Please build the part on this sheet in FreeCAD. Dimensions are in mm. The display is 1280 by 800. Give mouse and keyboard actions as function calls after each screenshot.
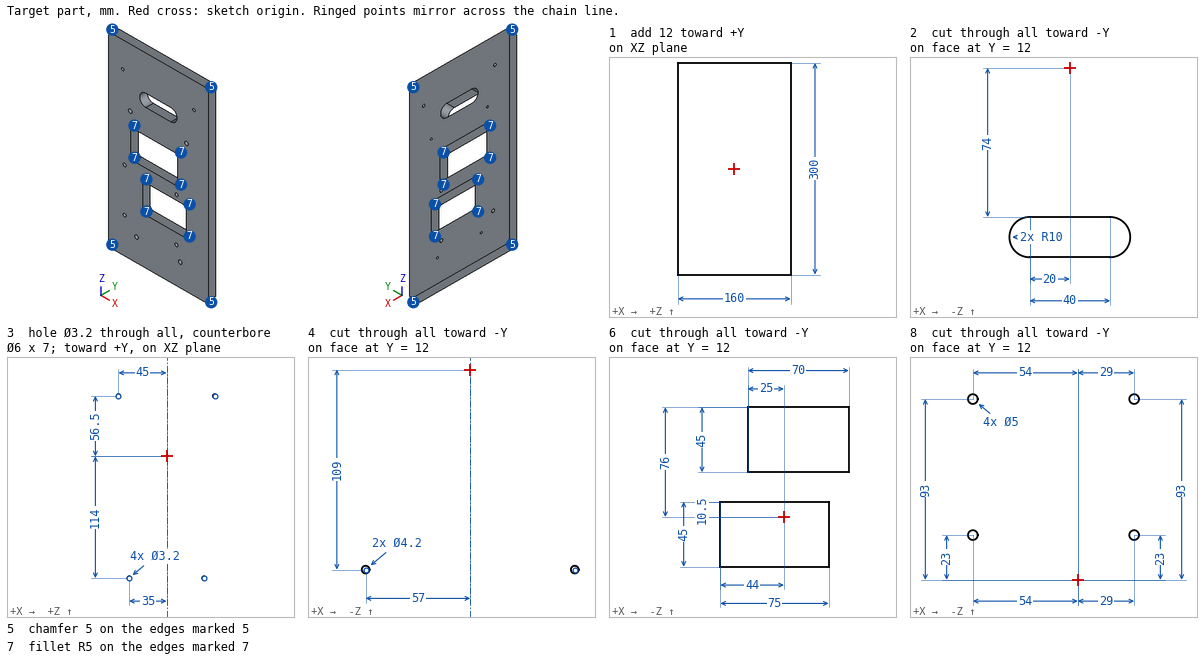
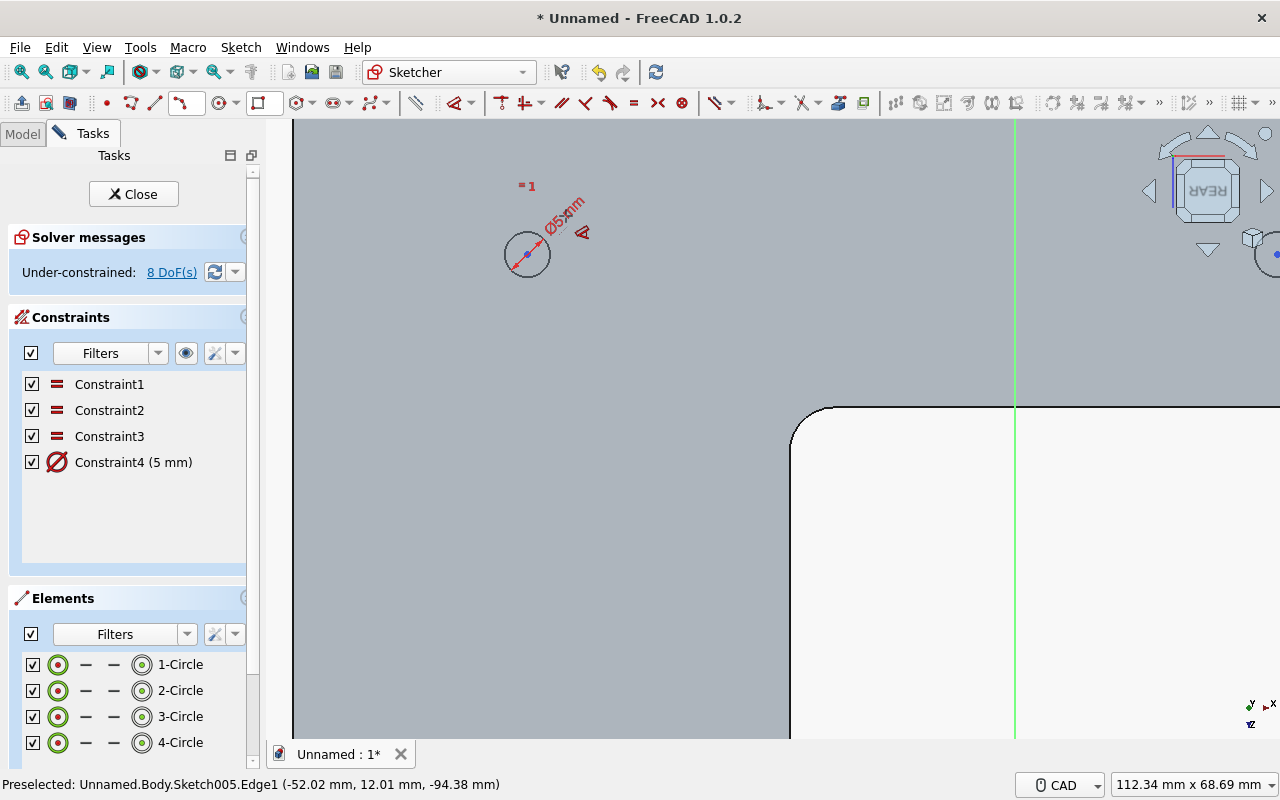
click(527, 255)
click(771, 221)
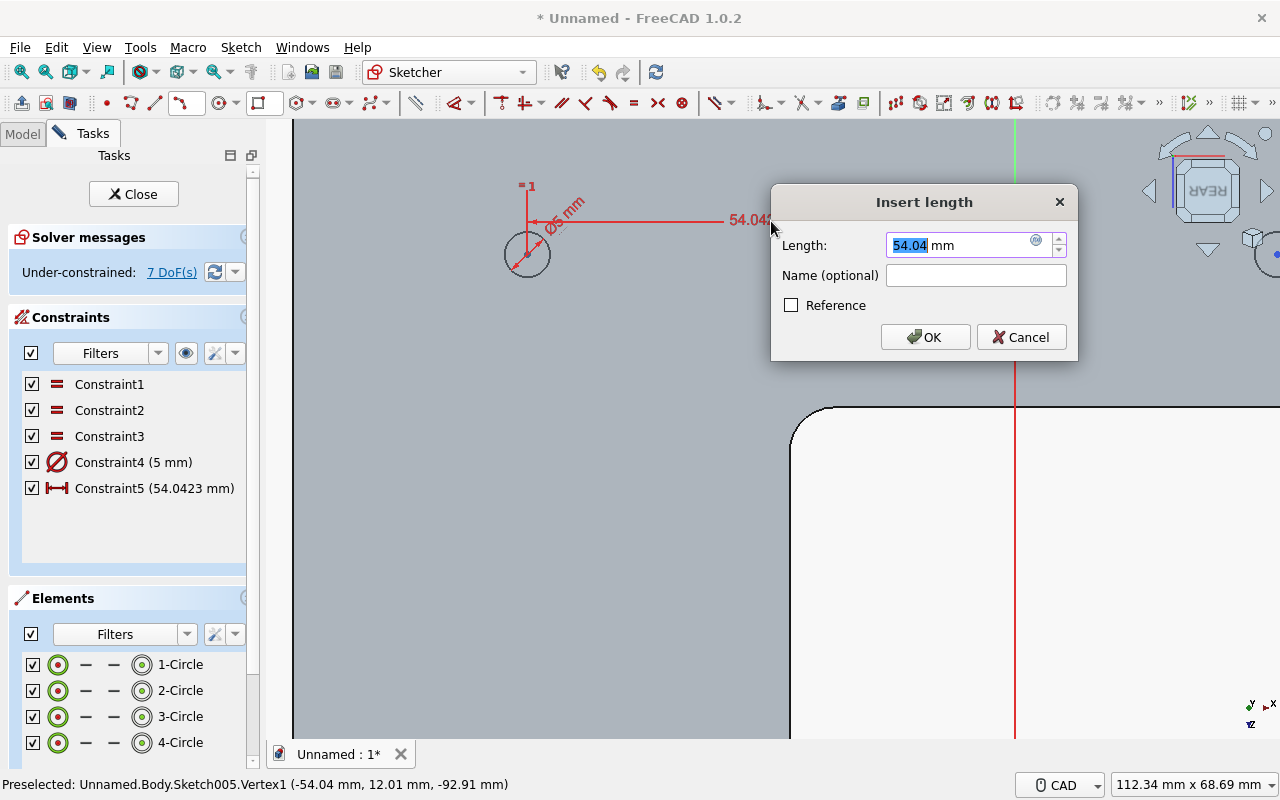
text(54)
key(Return)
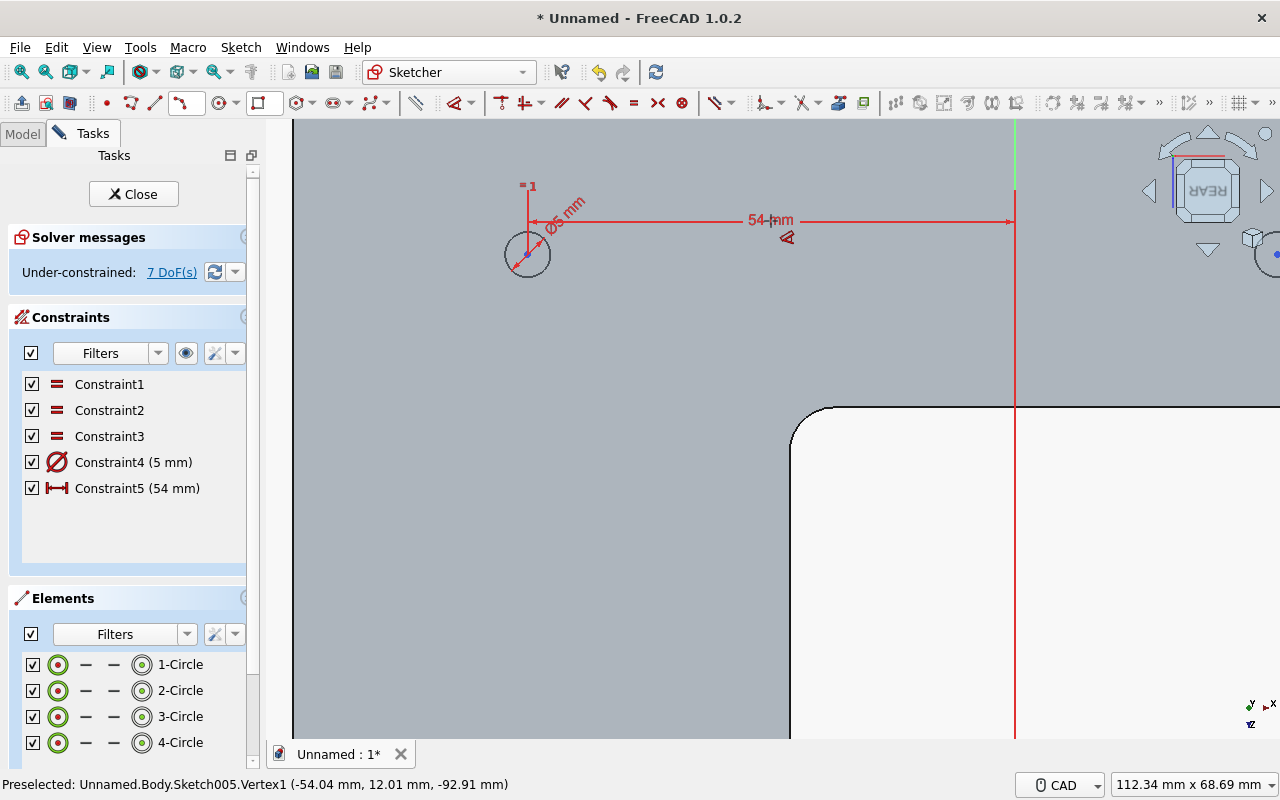
click(528, 255)
click(494, 483)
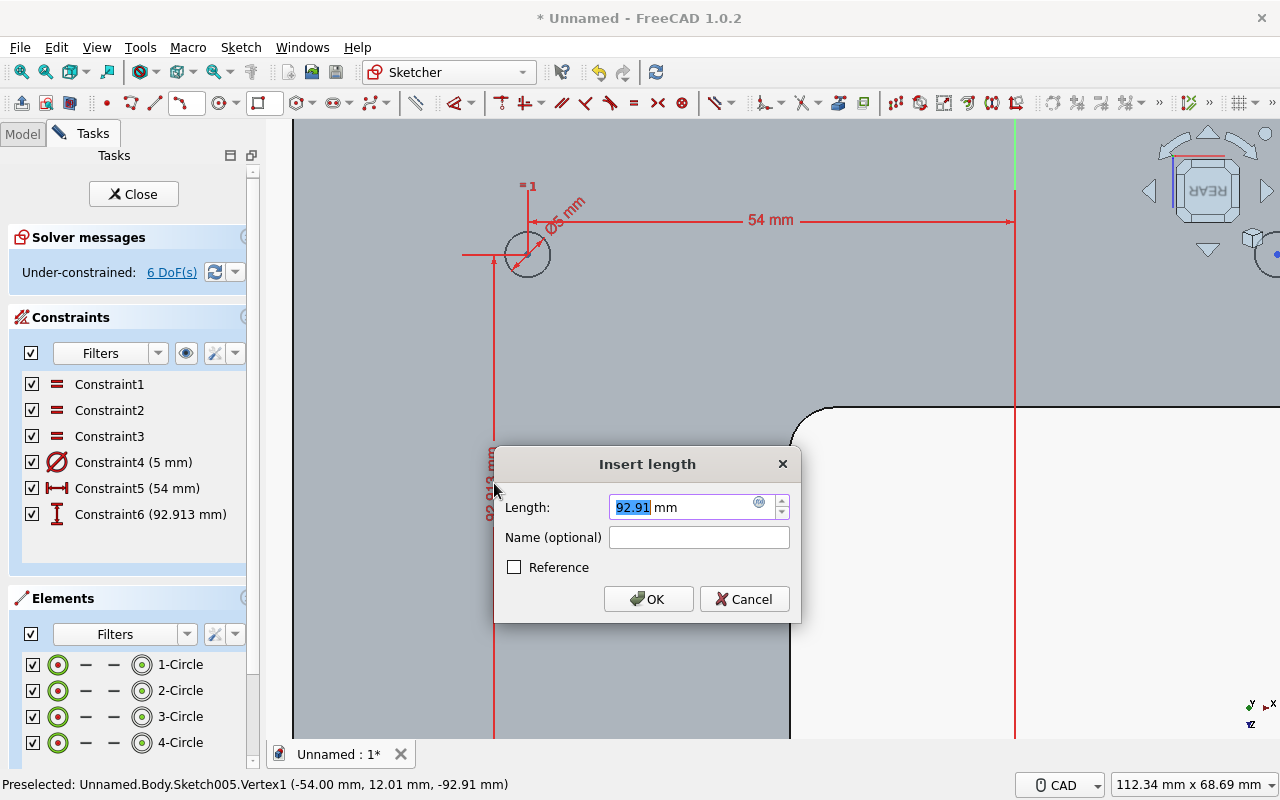
text(93)
key(Return)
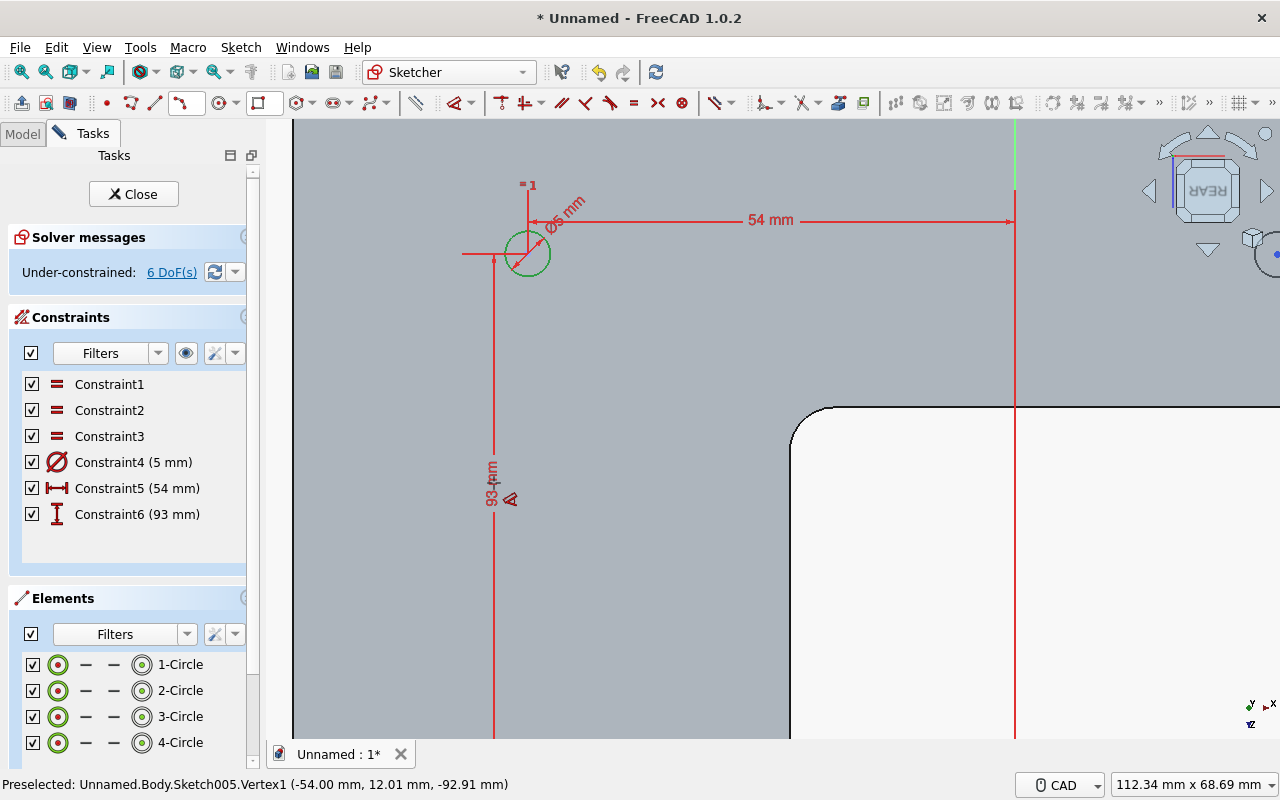
scroll(543, 239, down, 4)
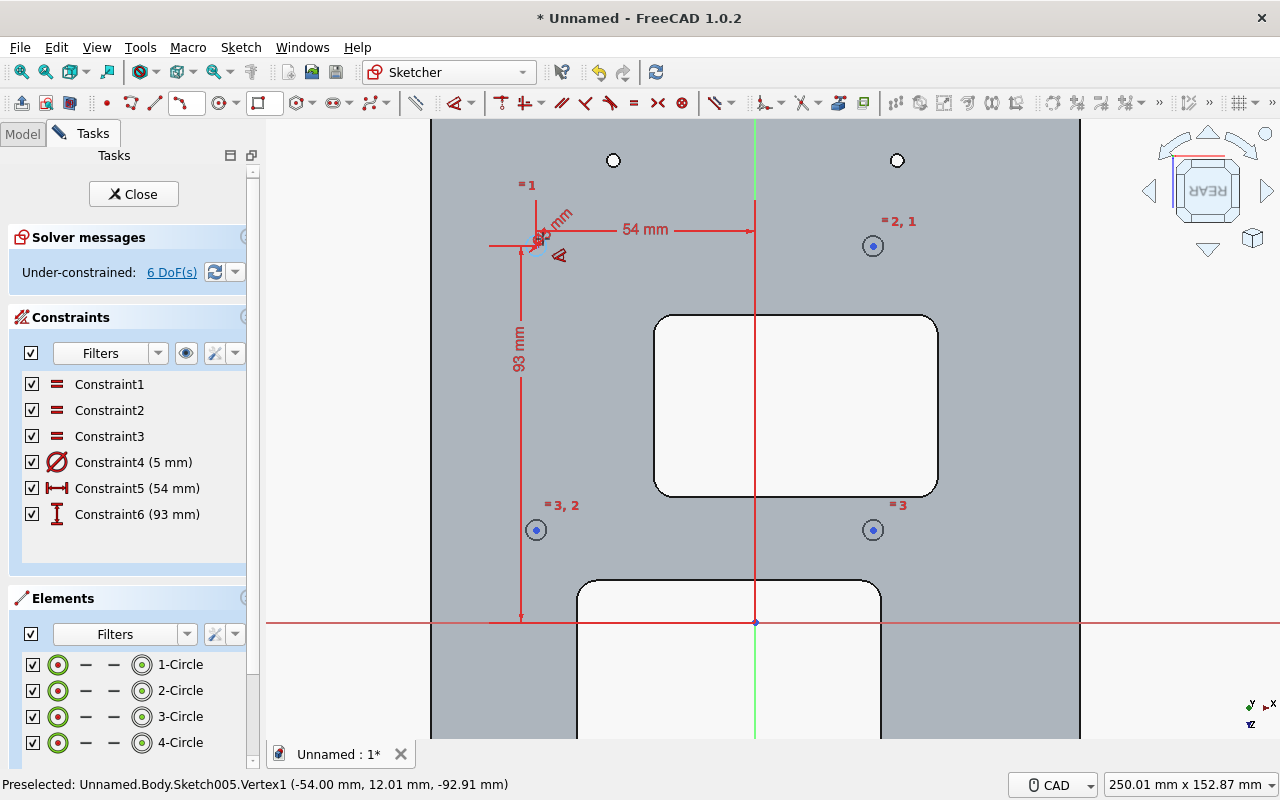
click(873, 246)
click(814, 657)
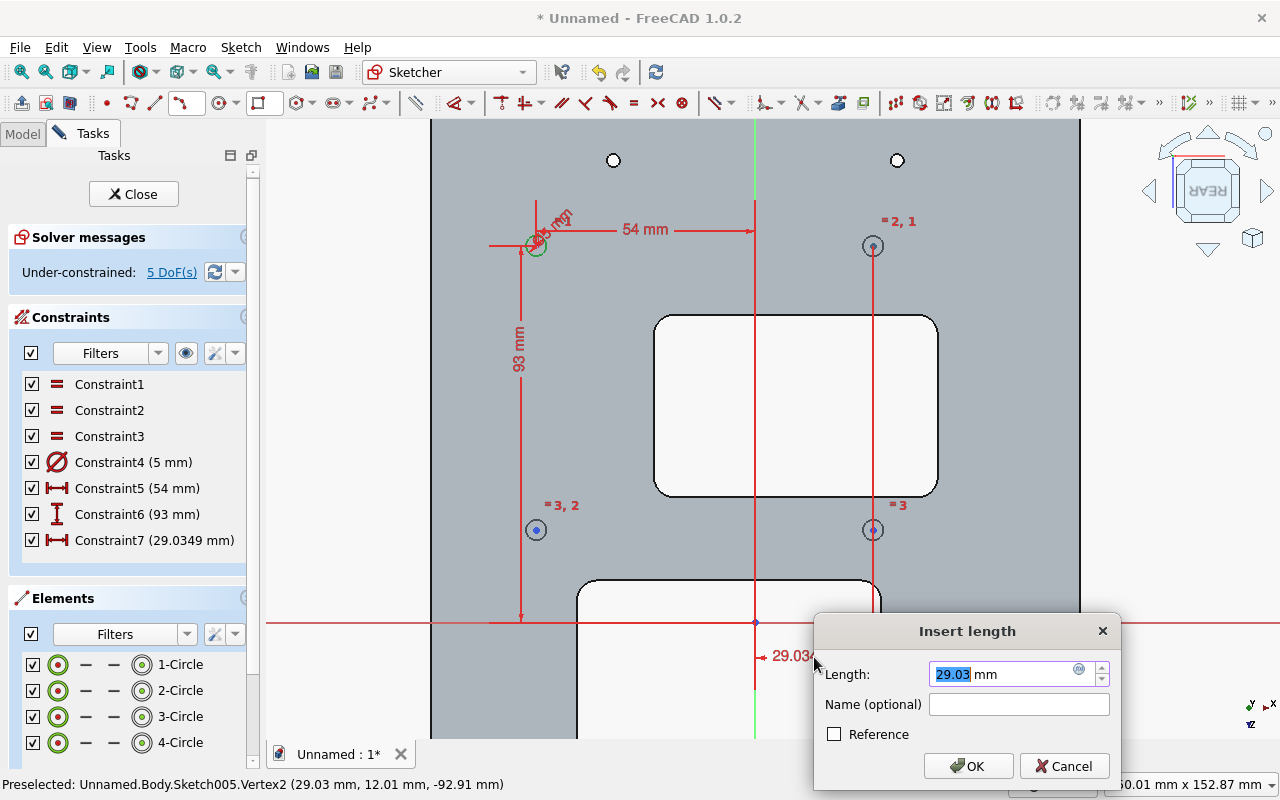
text(29)
key(Return)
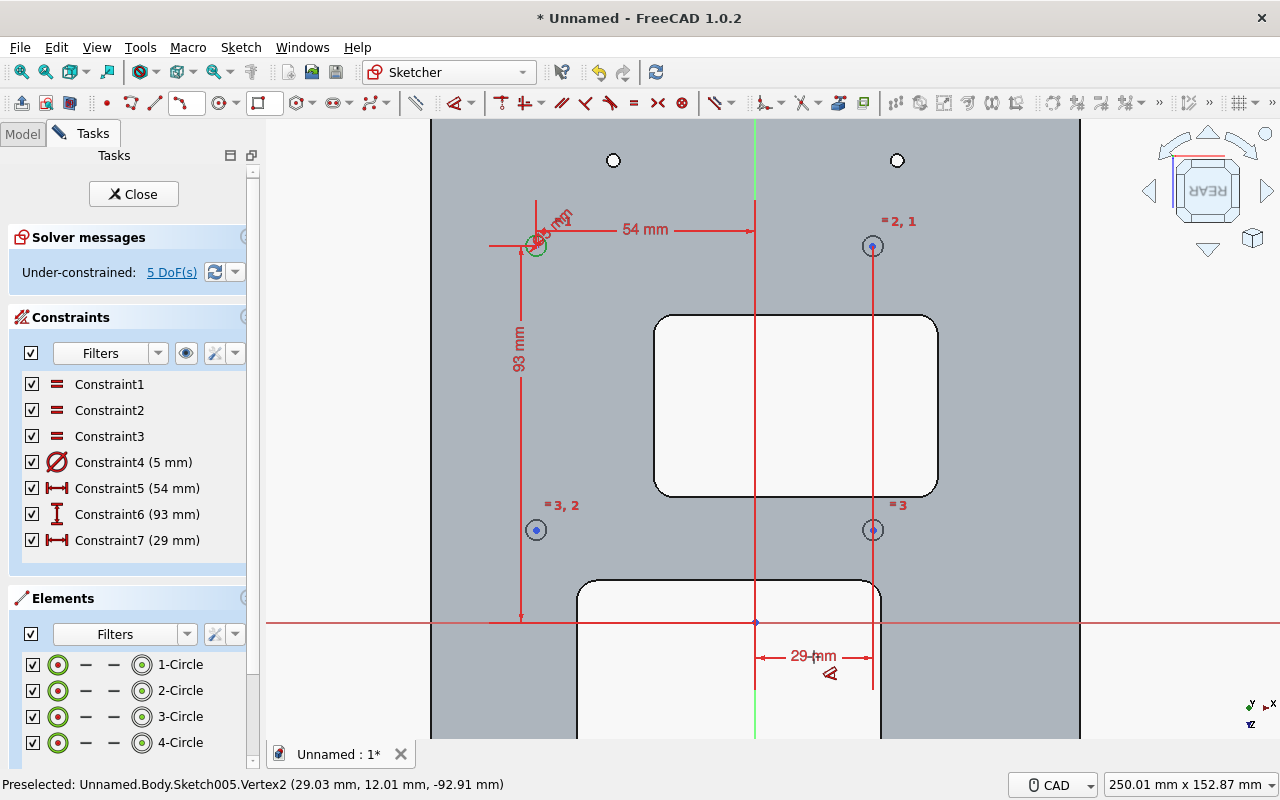
click(873, 246)
click(907, 435)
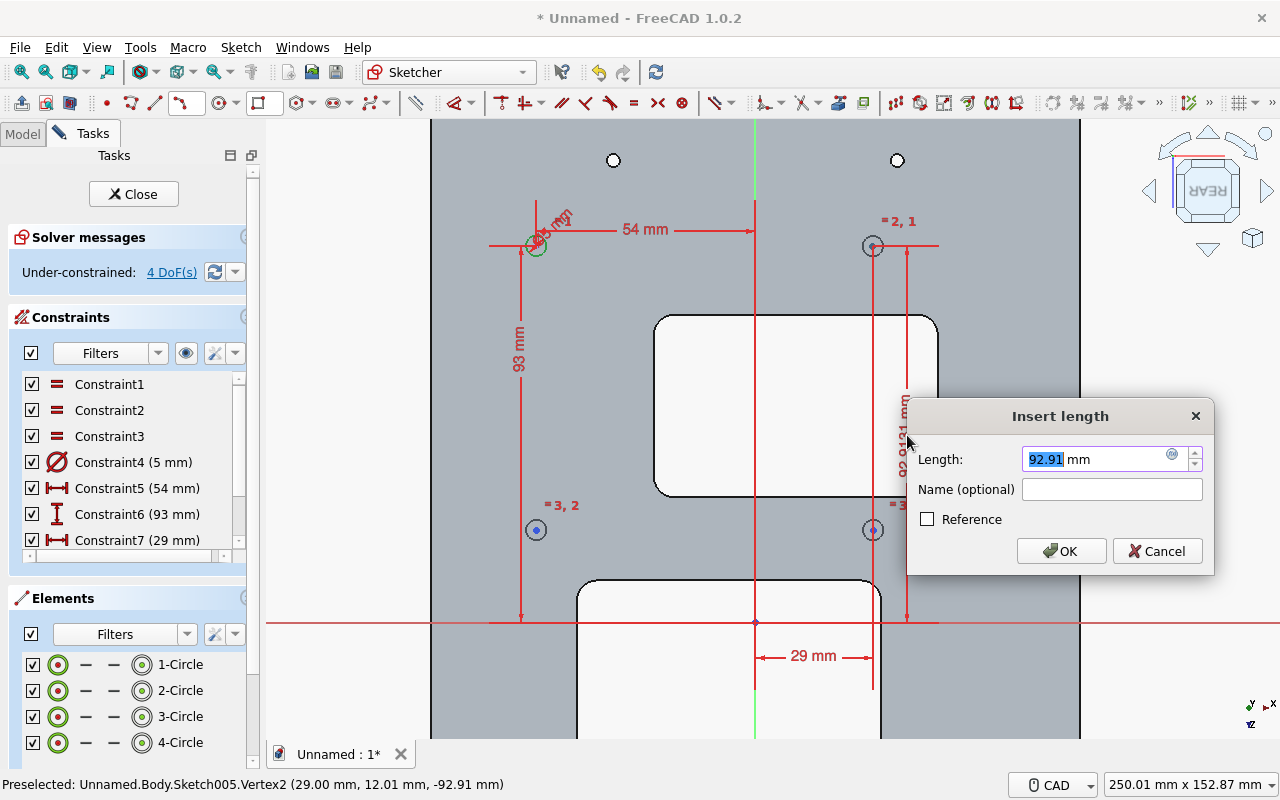
text(93)
key(Return)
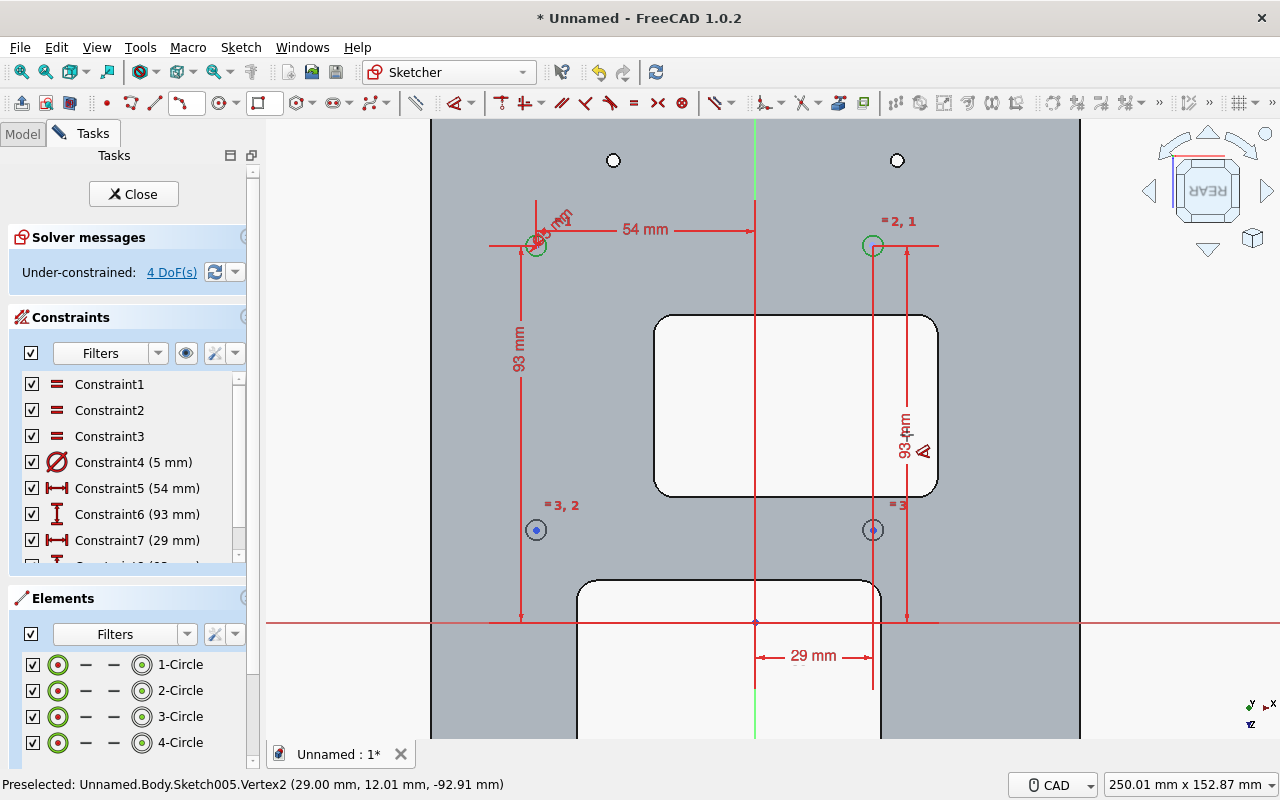
click(536, 530)
click(646, 657)